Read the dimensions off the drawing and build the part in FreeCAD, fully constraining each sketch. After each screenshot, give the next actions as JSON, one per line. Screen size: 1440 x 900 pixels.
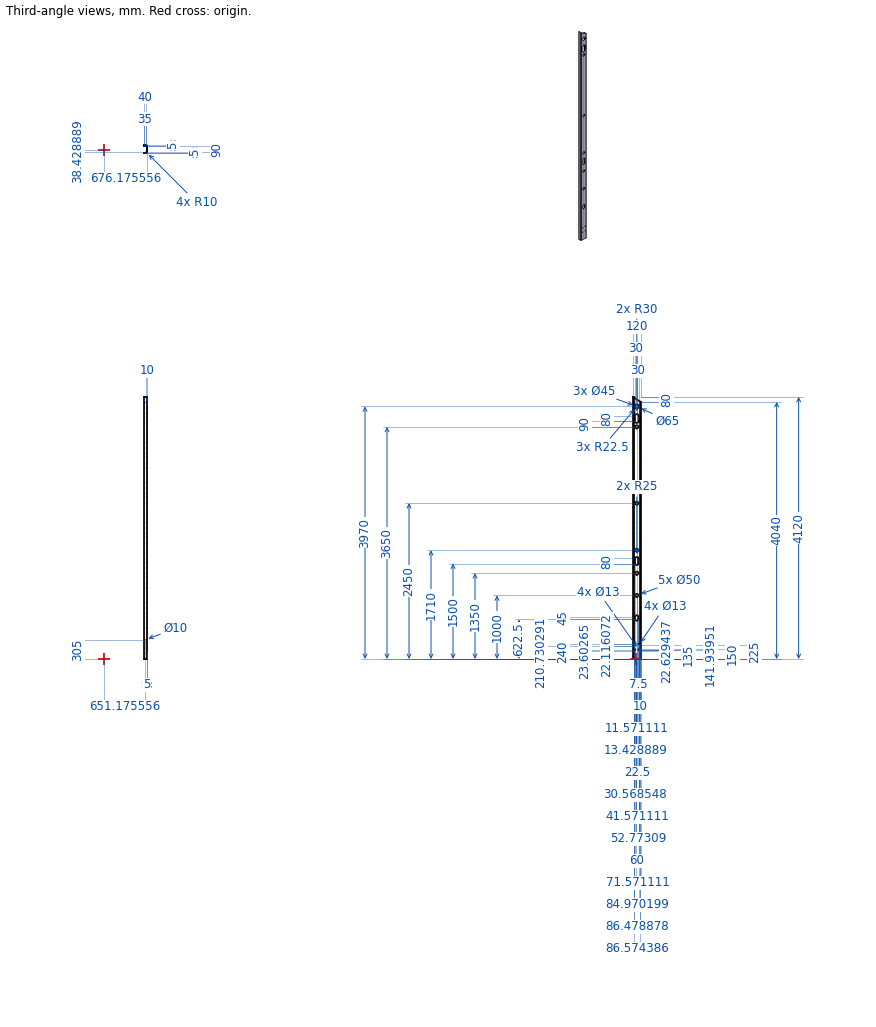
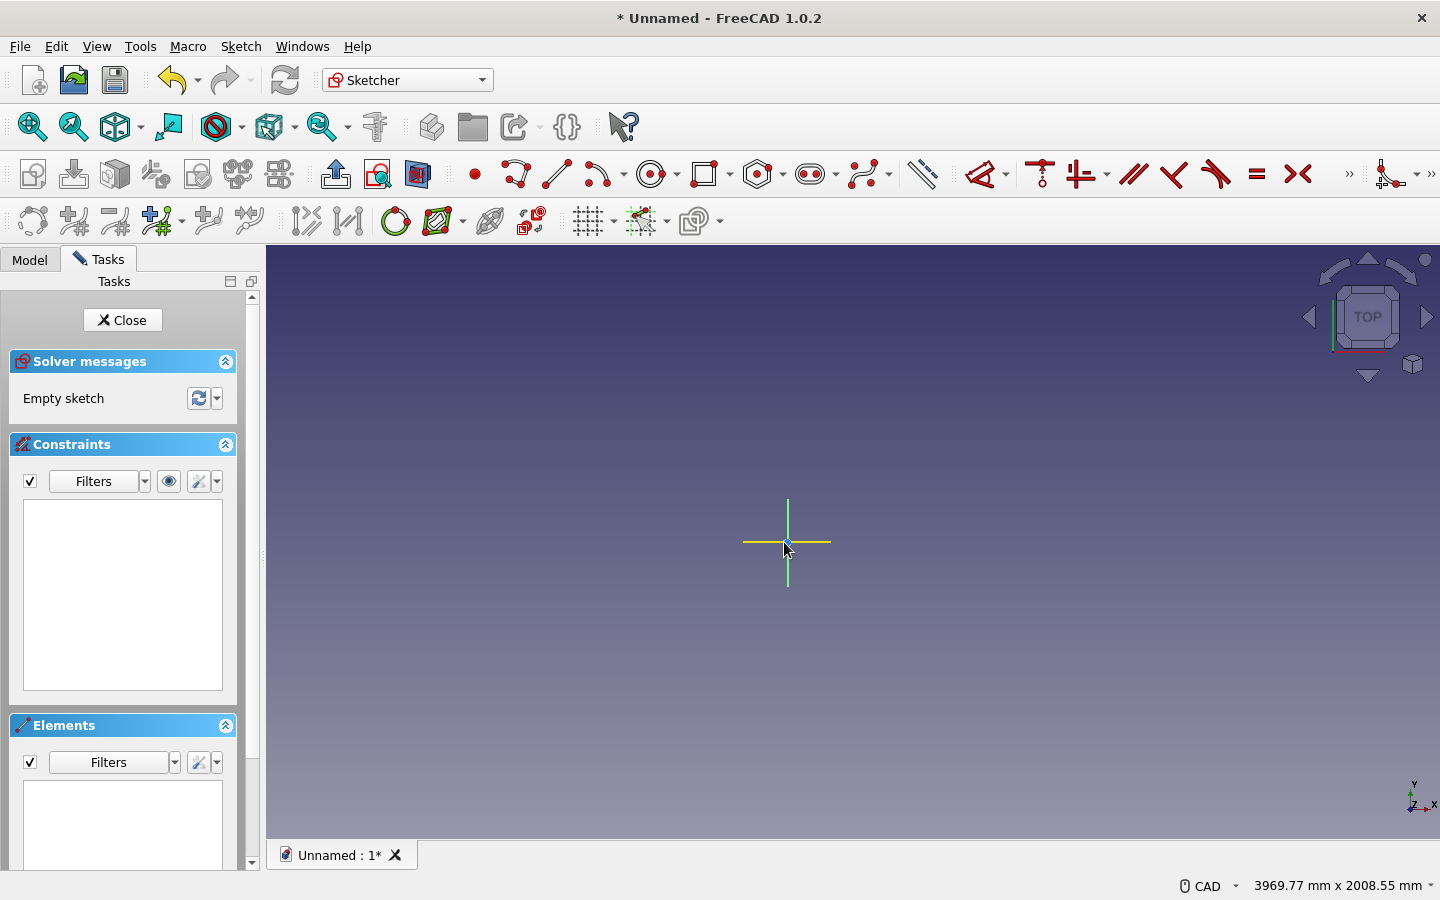
{"action": "scroll", "coordinate": [1000, 539], "scroll_direction": "up", "scroll_amount": 12}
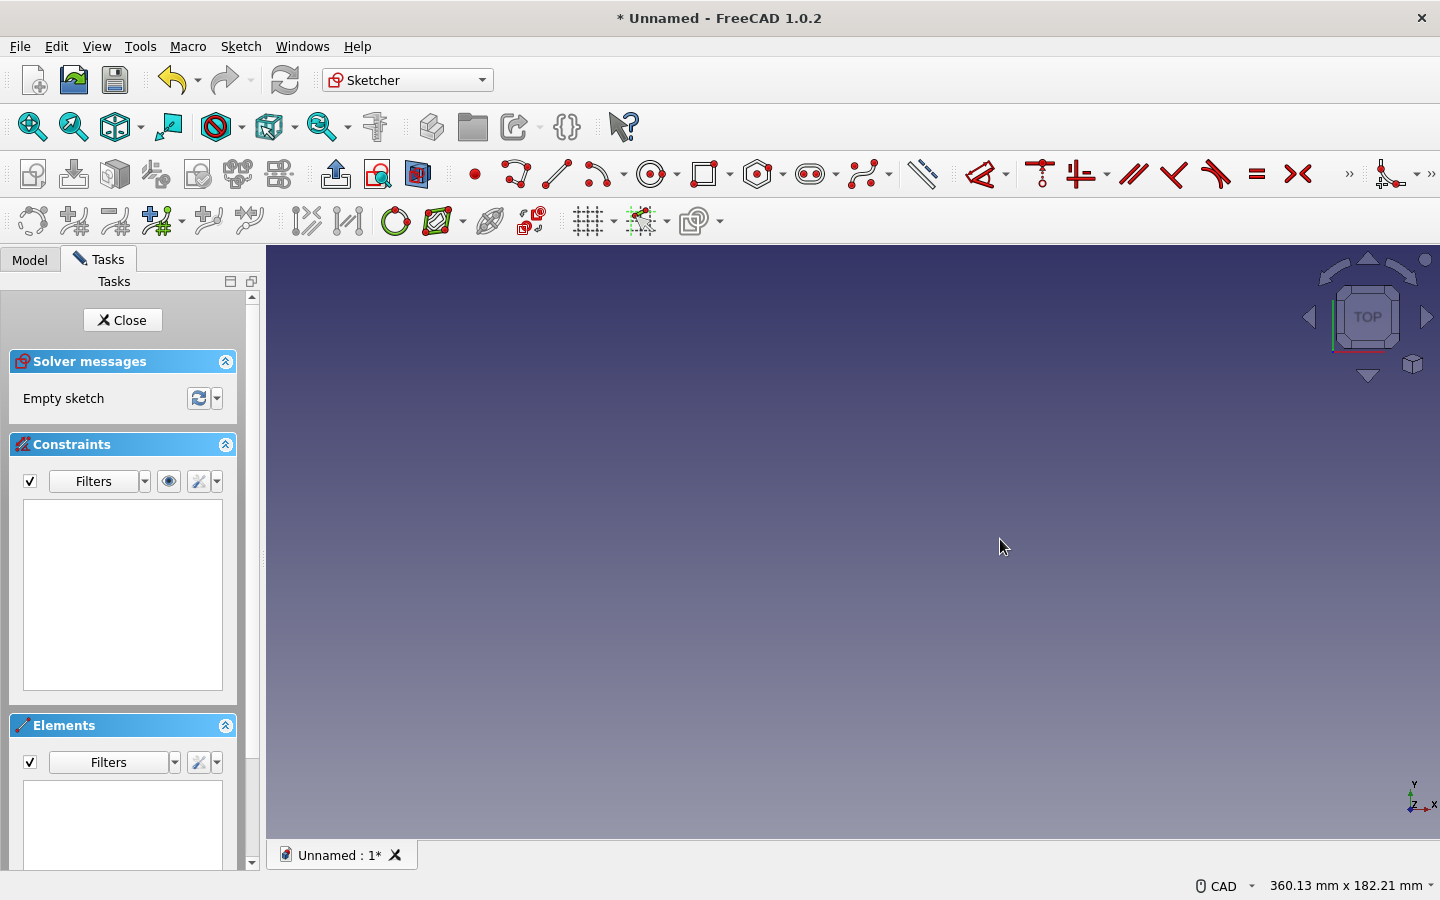
{"action": "left_click", "coordinate": [557, 174]}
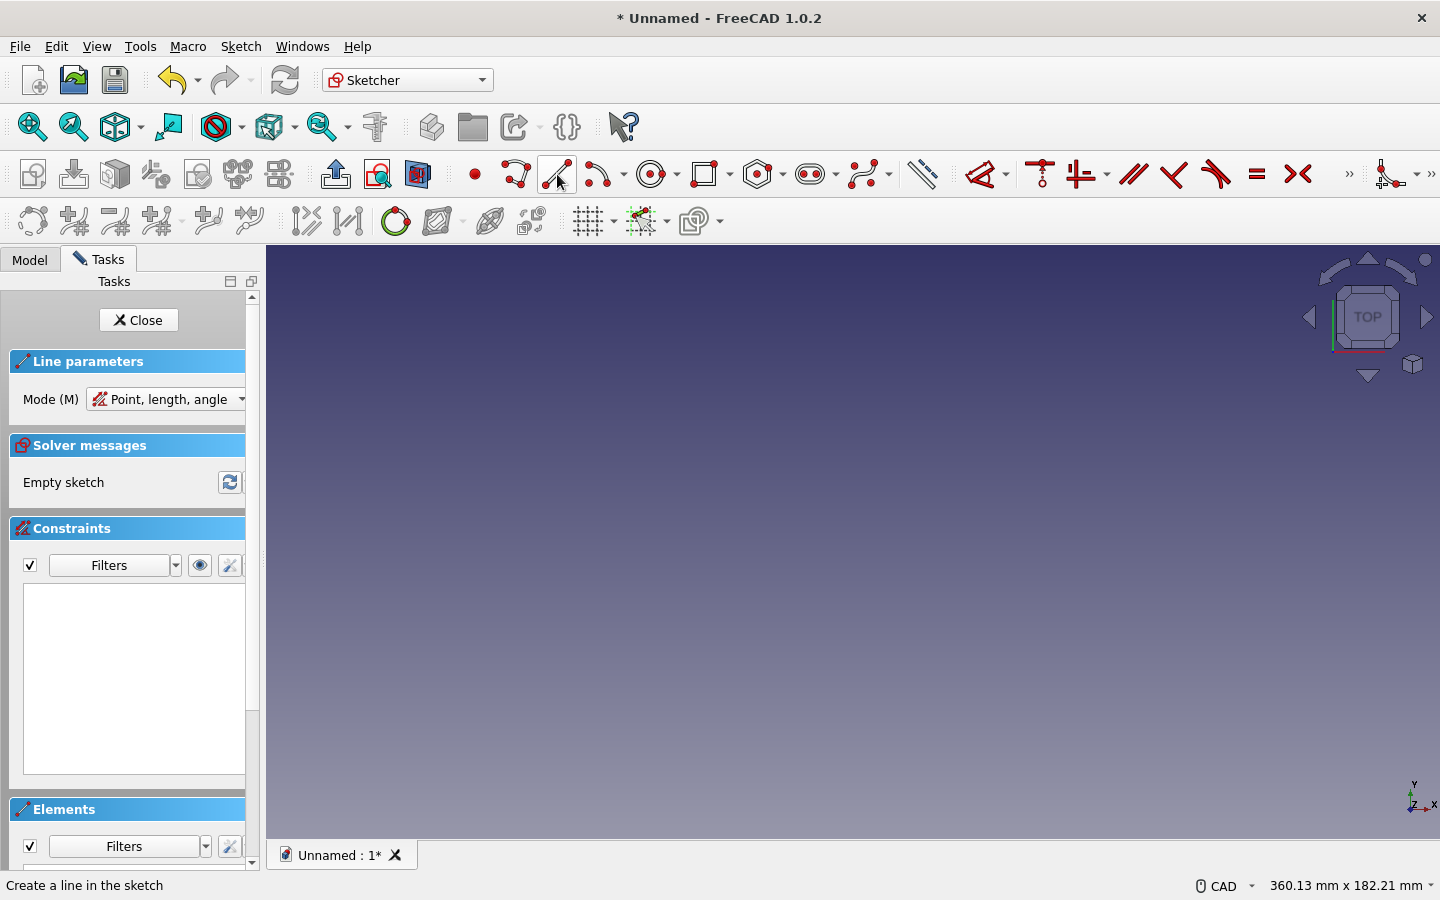
{"action": "left_click", "coordinate": [860, 698]}
{"action": "left_click", "coordinate": [860, 372]}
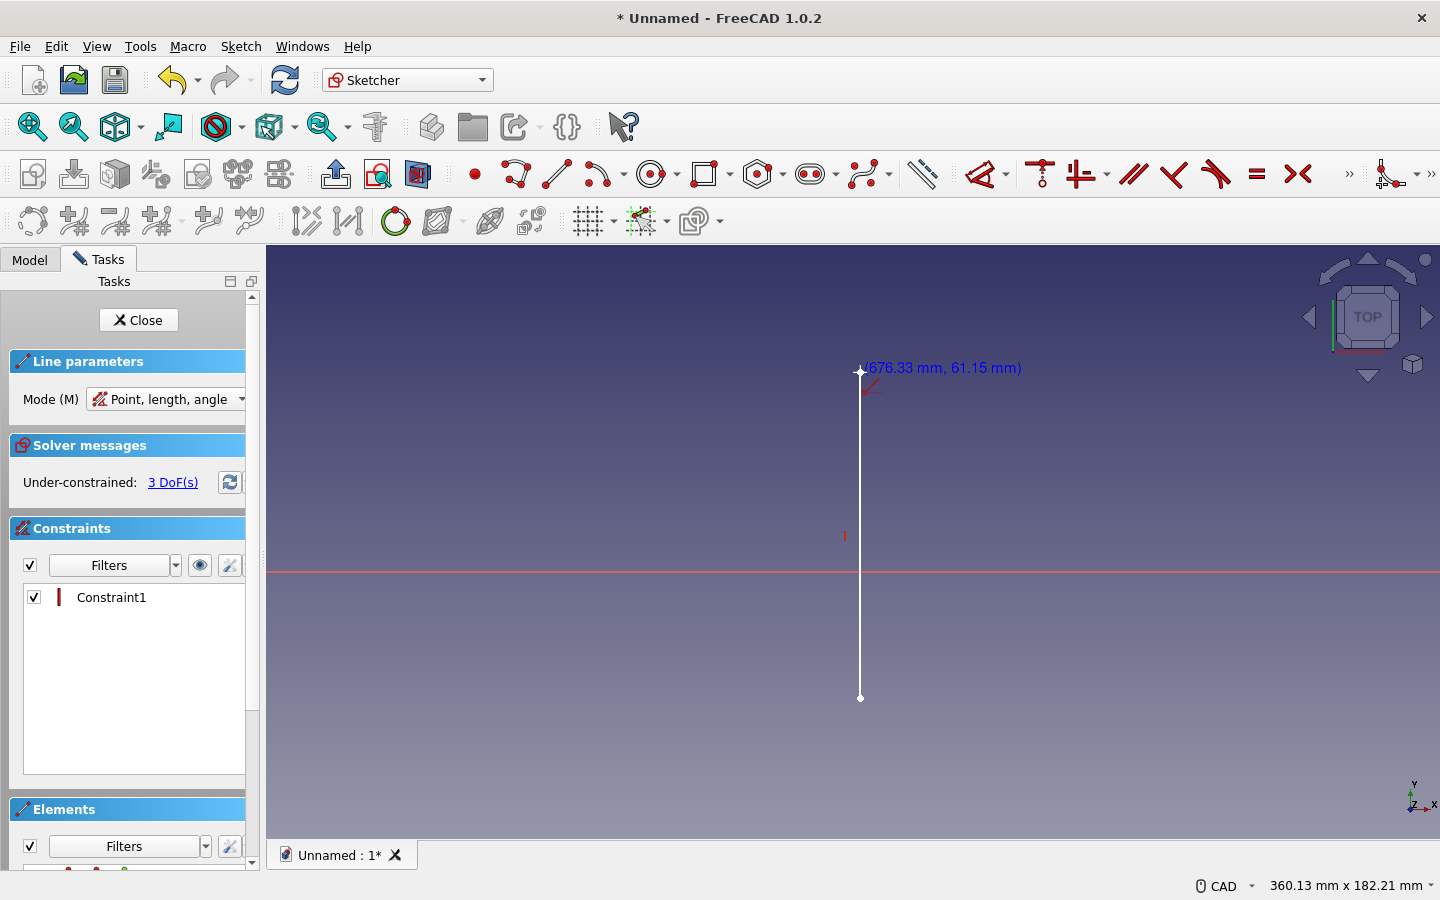
{"action": "key", "text": "g m"}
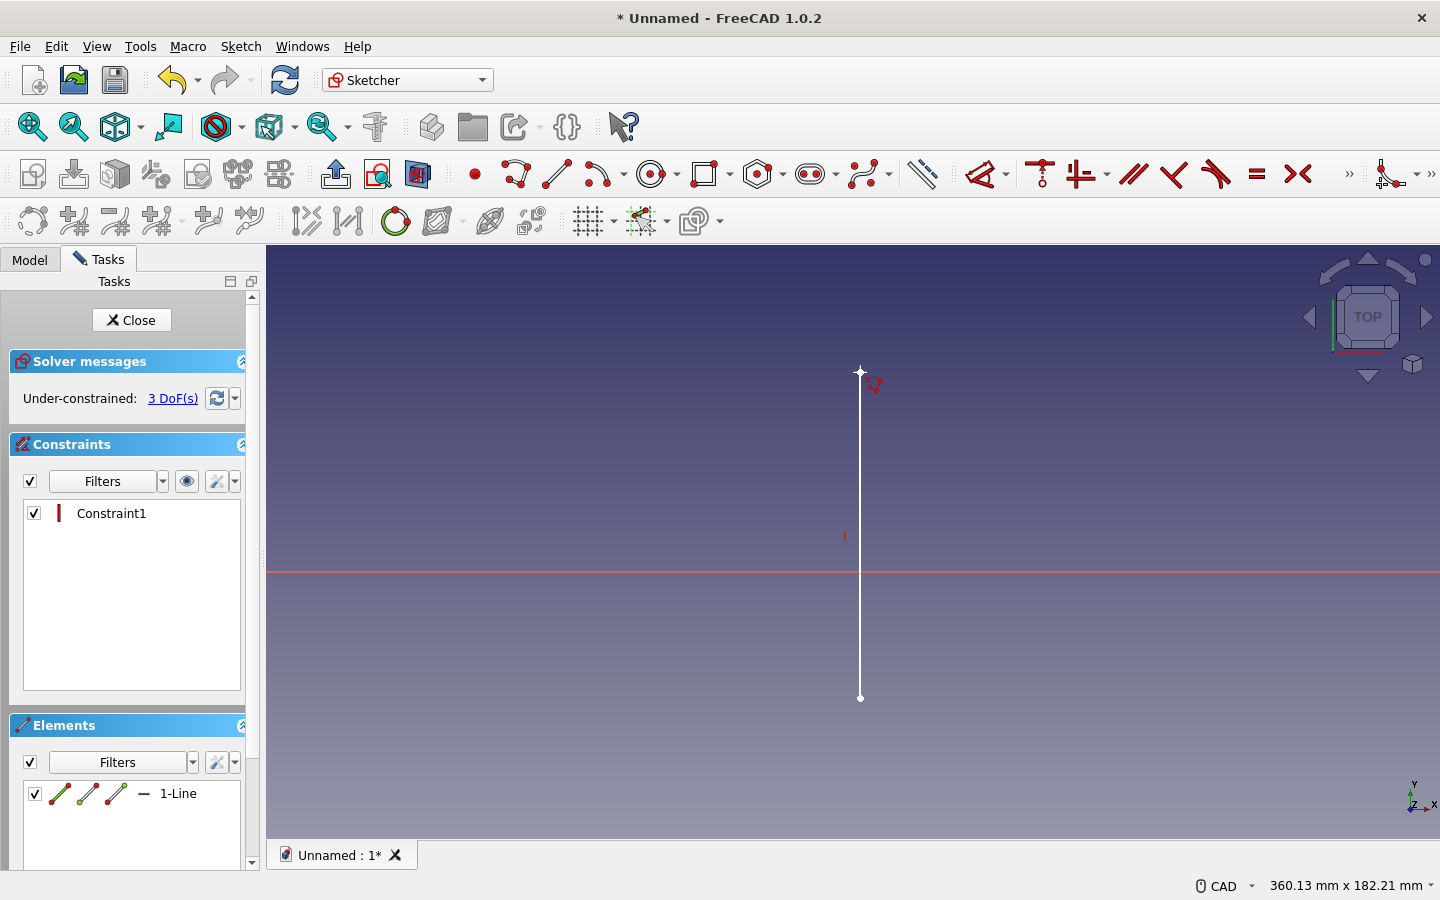
{"action": "left_click", "coordinate": [827, 339]}
{"action": "left_click", "coordinate": [697, 339]}
{"action": "left_click", "coordinate": [697, 355]}
{"action": "left_click", "coordinate": [811, 355]}
{"action": "right_click", "coordinate": [811, 355]}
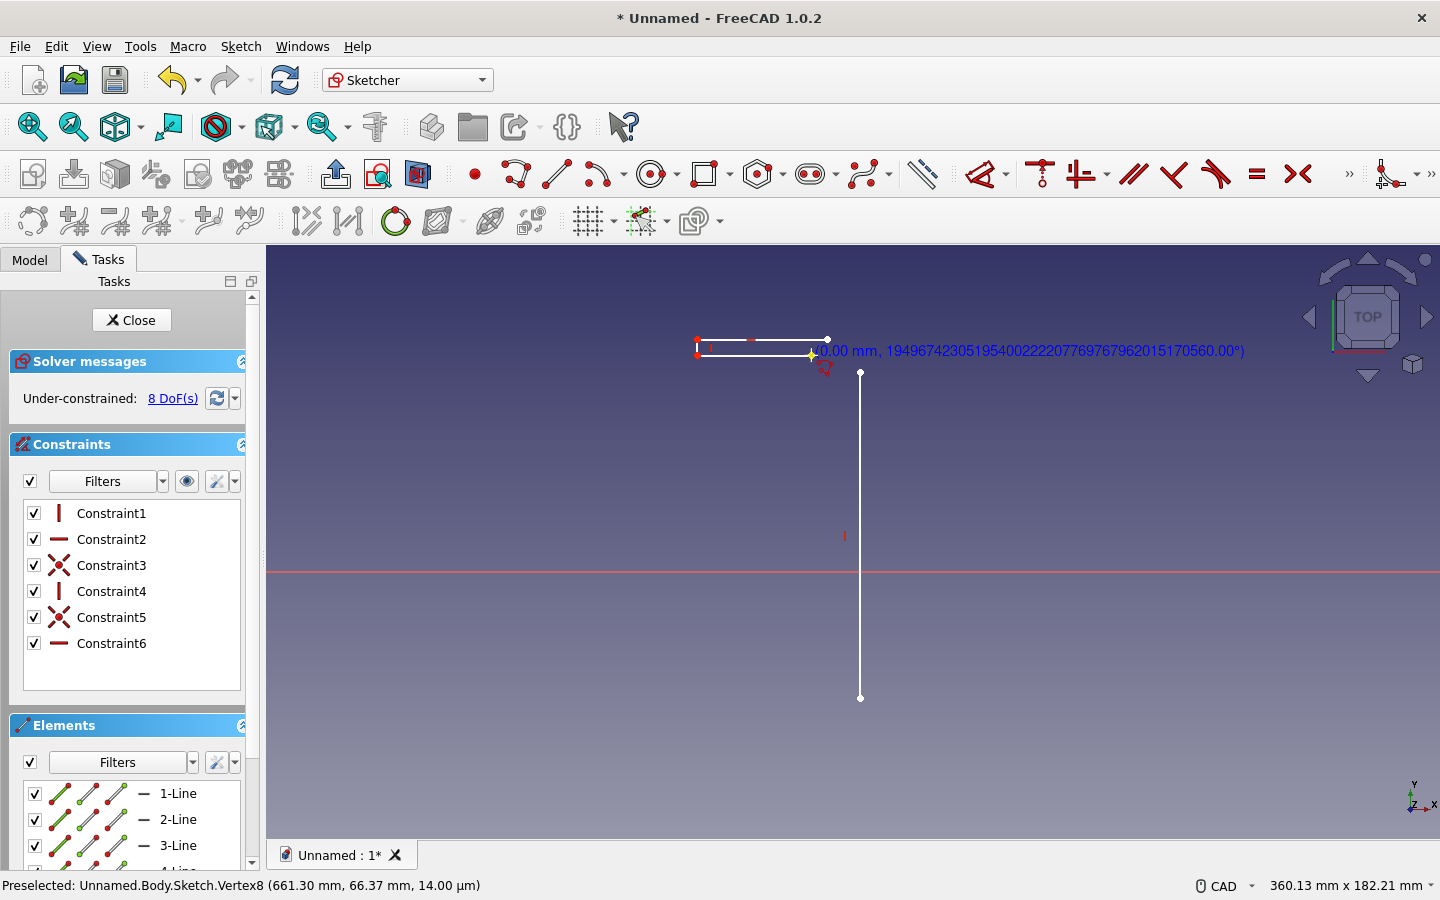
{"action": "key", "text": "g l"}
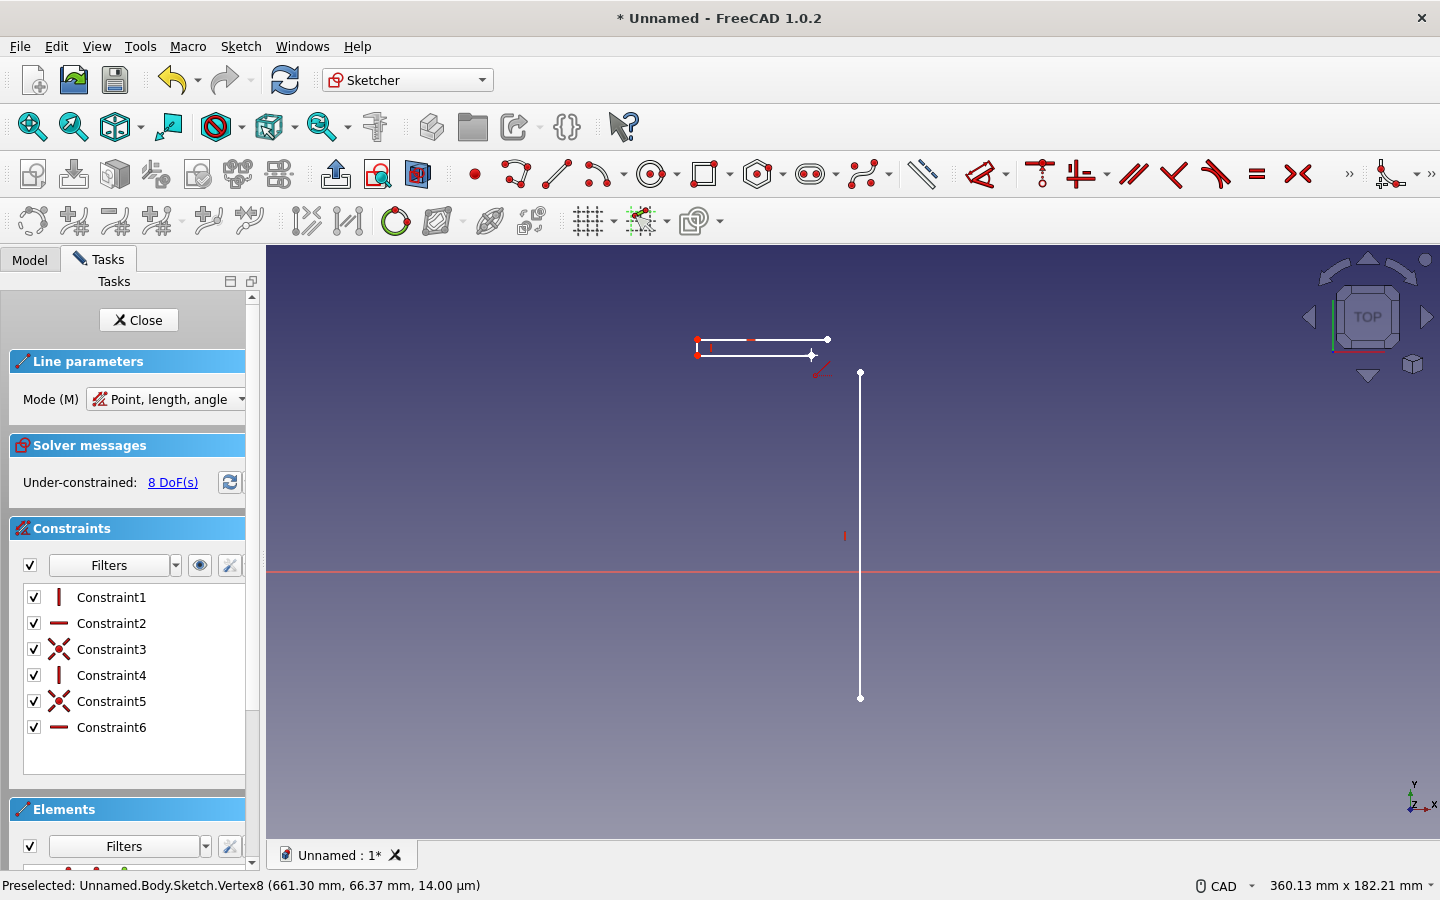
{"action": "left_click", "coordinate": [843, 388]}
{"action": "left_click", "coordinate": [843, 681]}